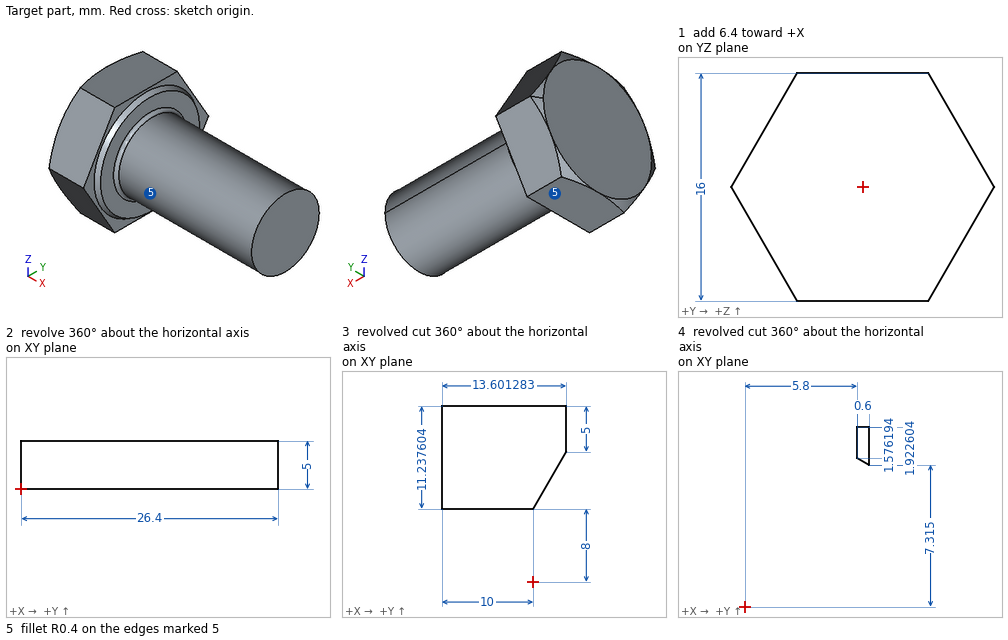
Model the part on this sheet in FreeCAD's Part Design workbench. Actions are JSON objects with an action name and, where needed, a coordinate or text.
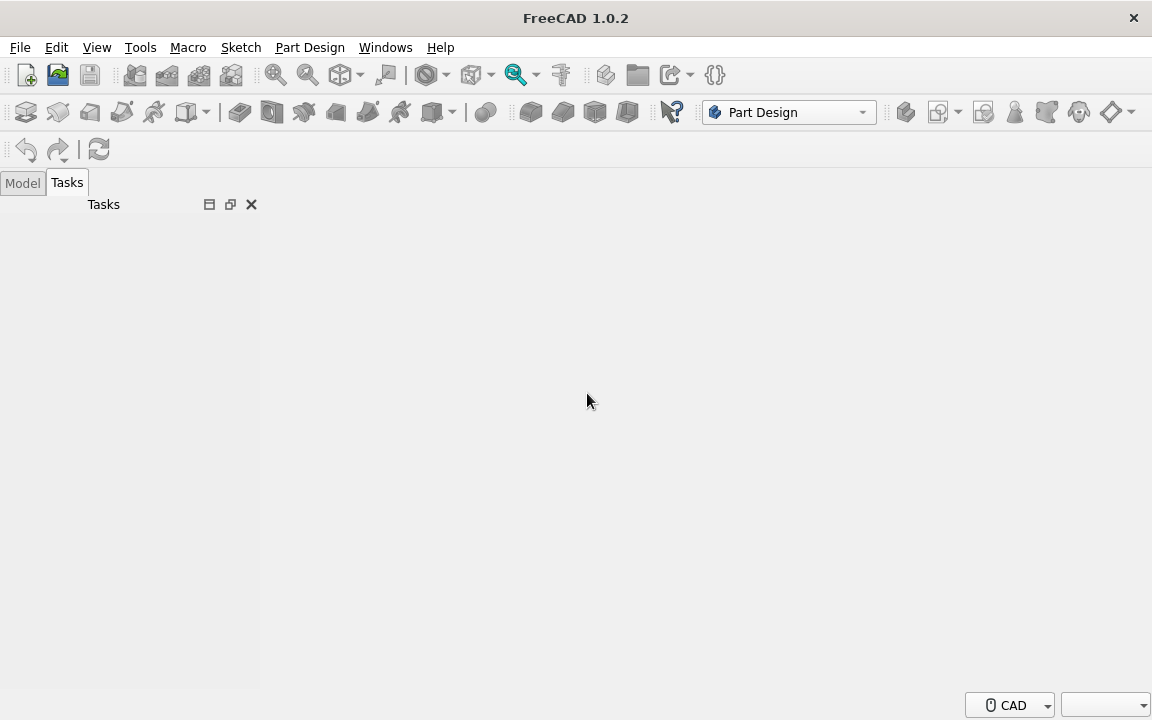
{"action": "left_click", "coordinate": [26, 76]}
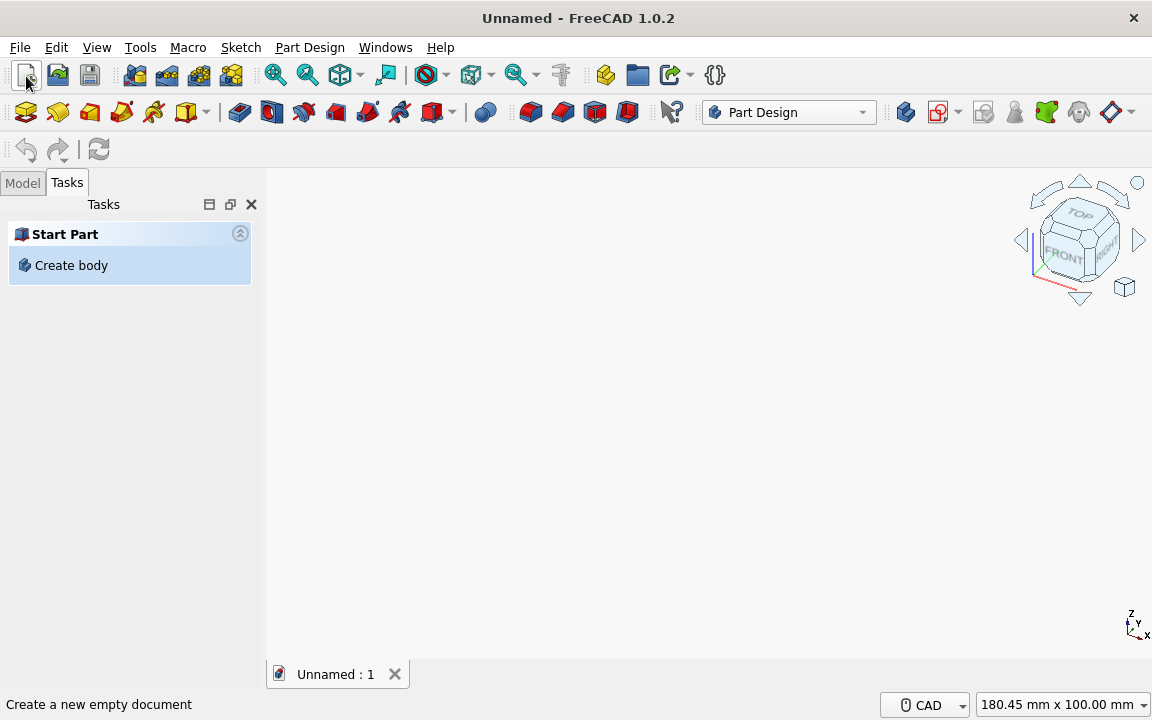
{"action": "left_click", "coordinate": [938, 112]}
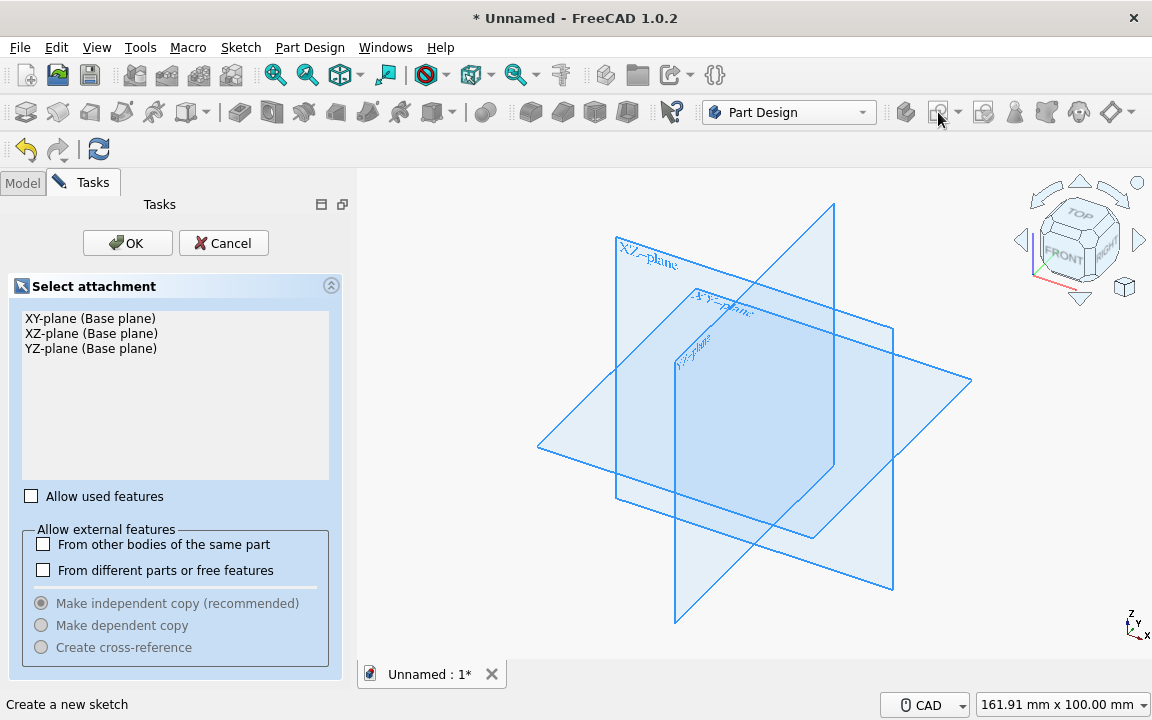
{"action": "left_click", "coordinate": [82, 348]}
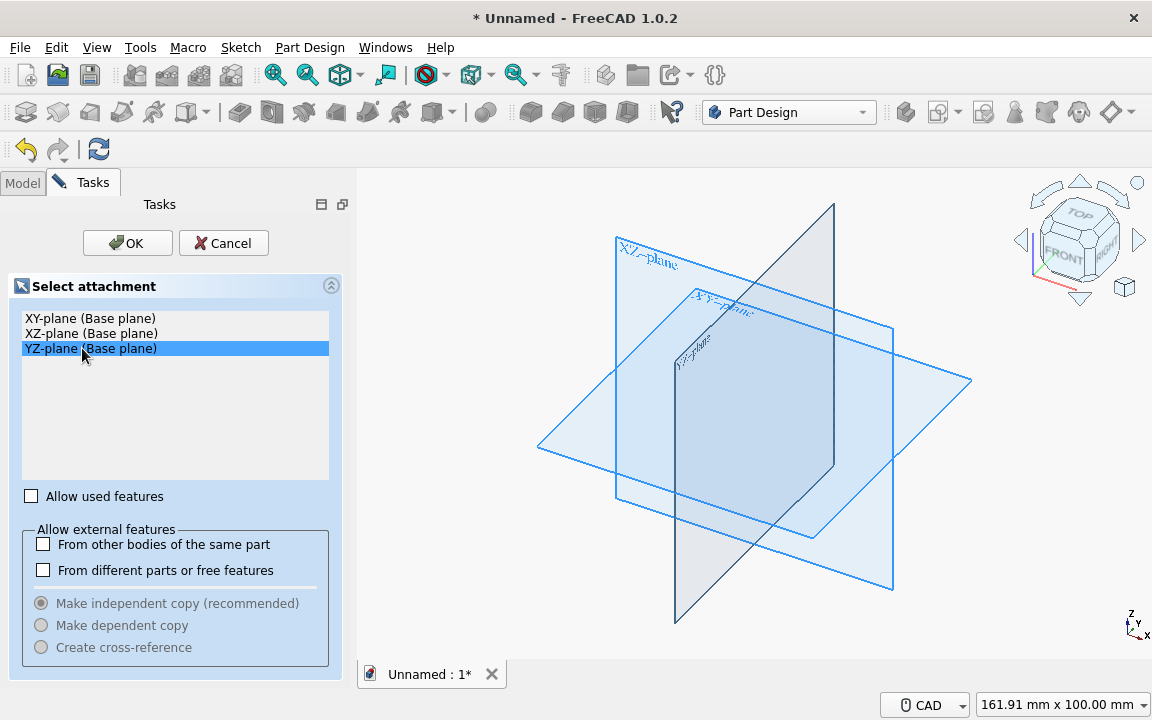
{"action": "left_click", "coordinate": [128, 243]}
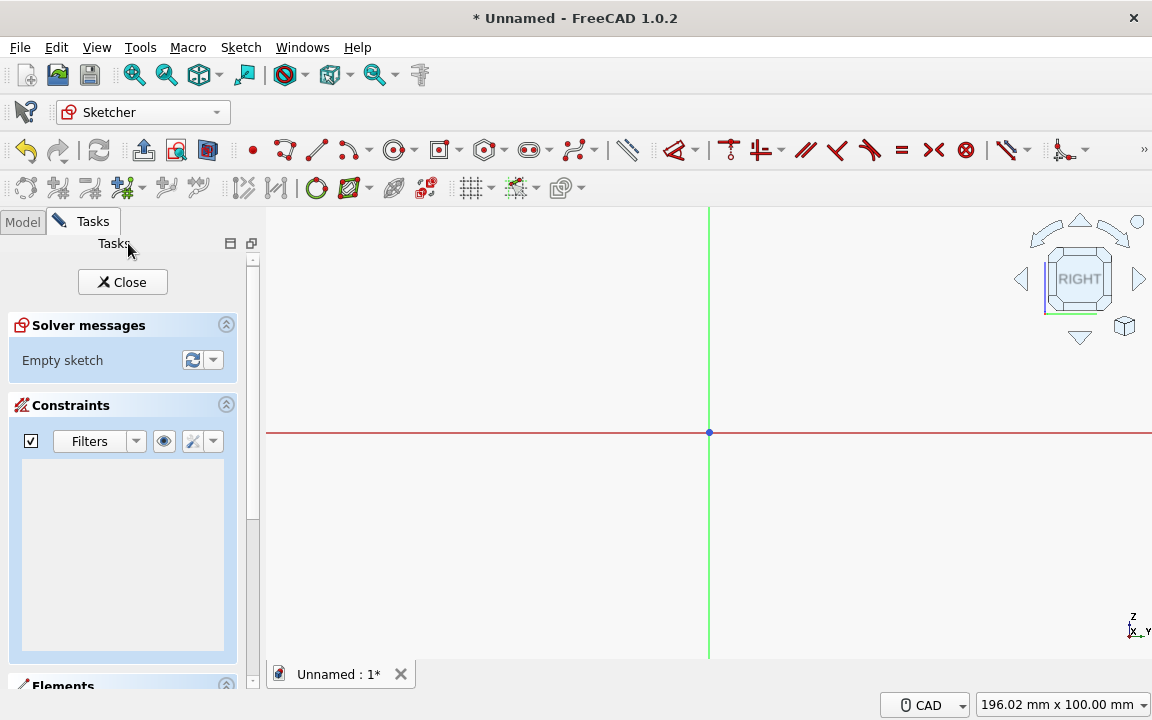
{"action": "scroll", "coordinate": [731, 433], "scroll_direction": "up", "scroll_amount": 7}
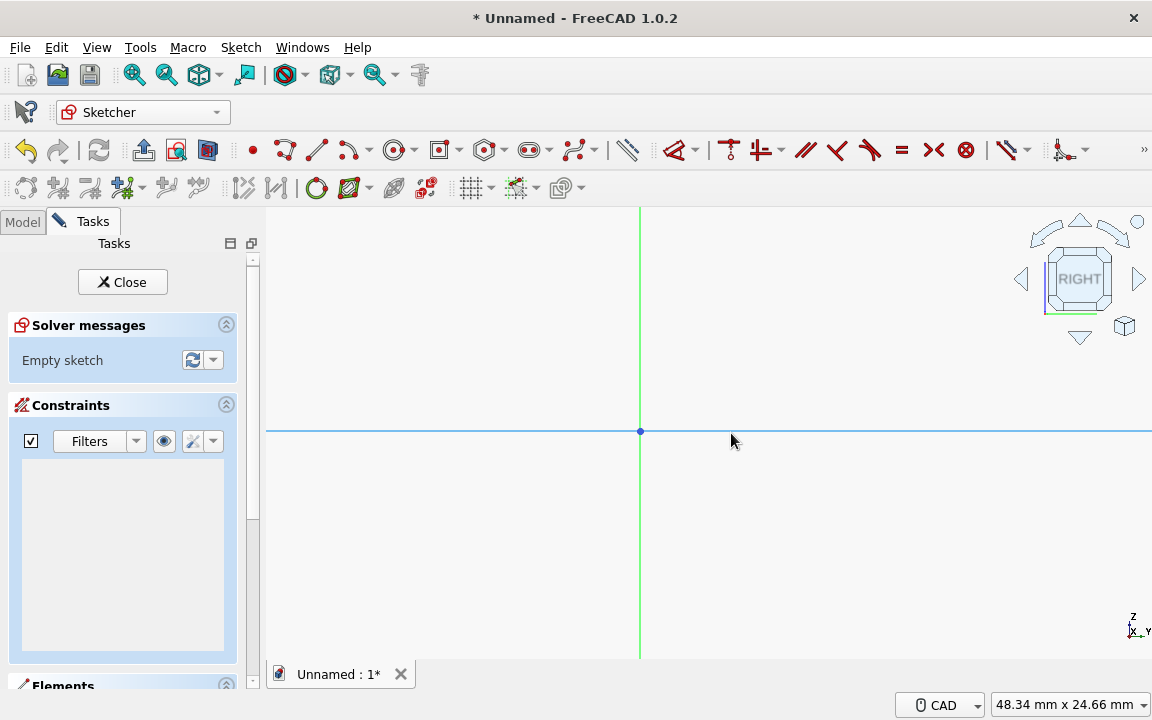
{"action": "left_click", "coordinate": [484, 150]}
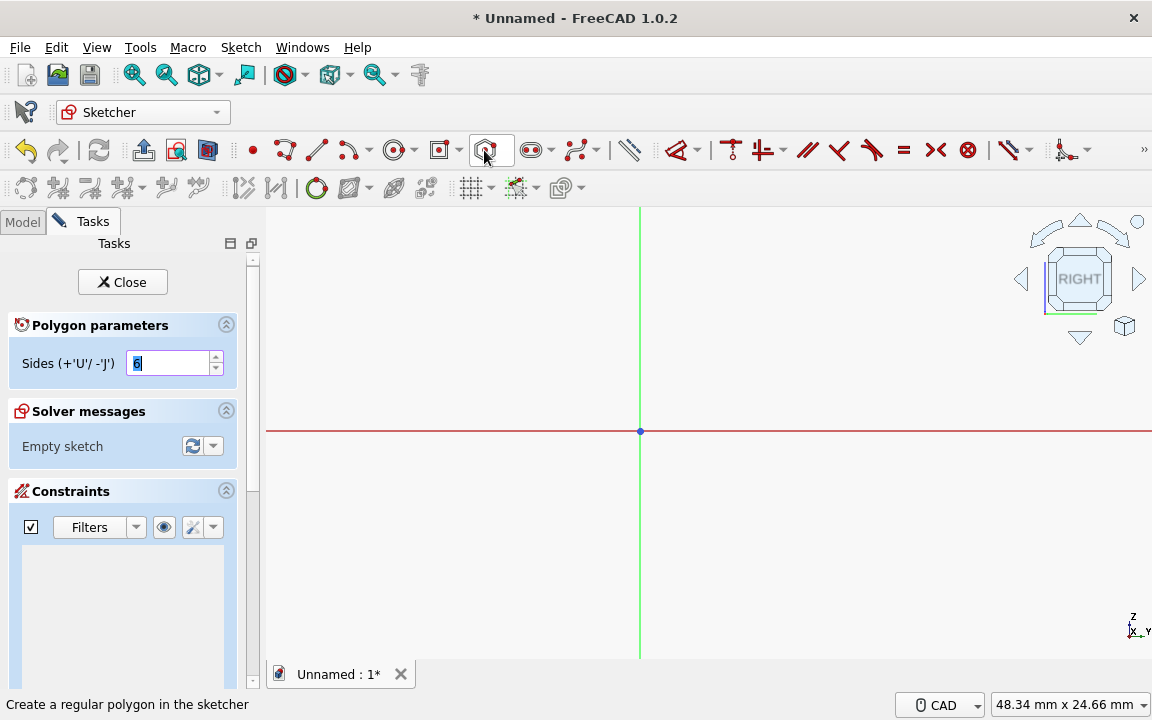
{"action": "left_click", "coordinate": [640, 431]}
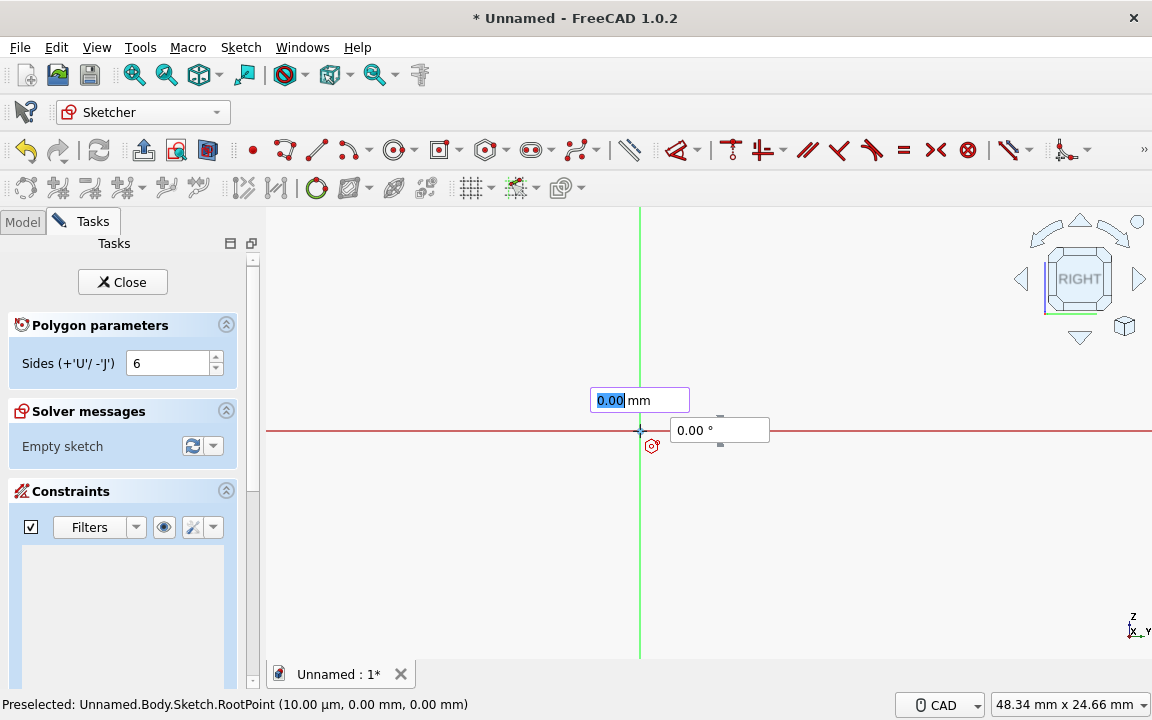
{"action": "left_click", "coordinate": [810, 431]}
{"action": "right_click", "coordinate": [810, 431]}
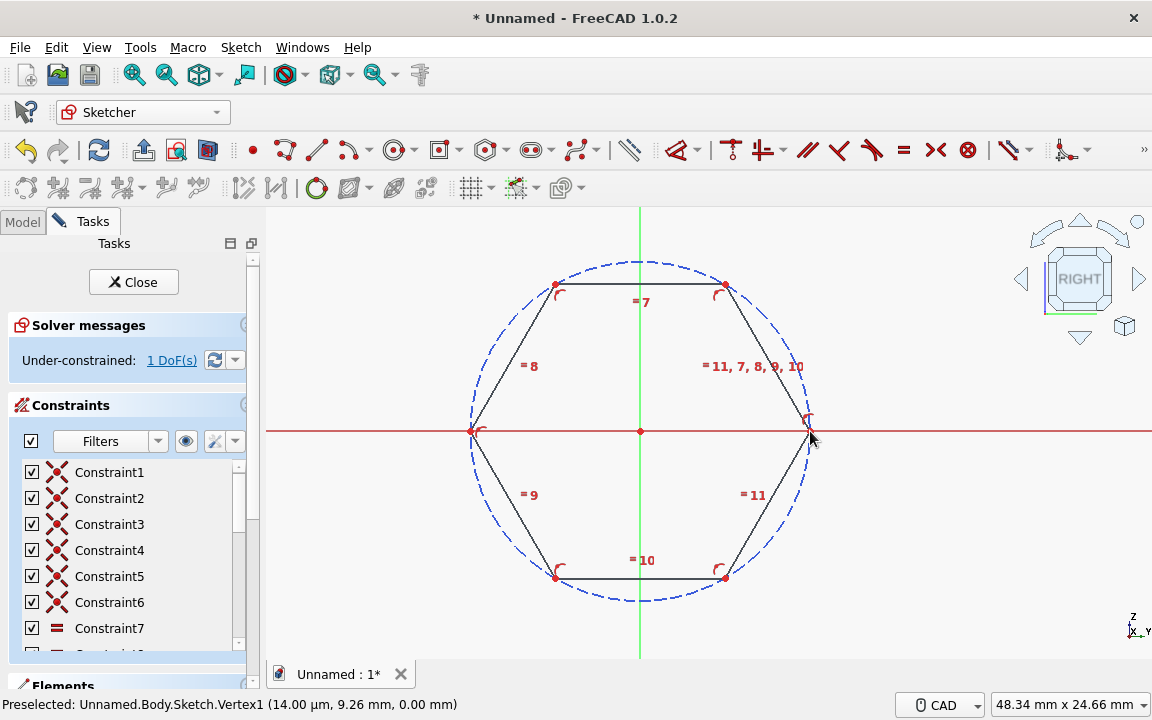
{"action": "left_click", "coordinate": [676, 150]}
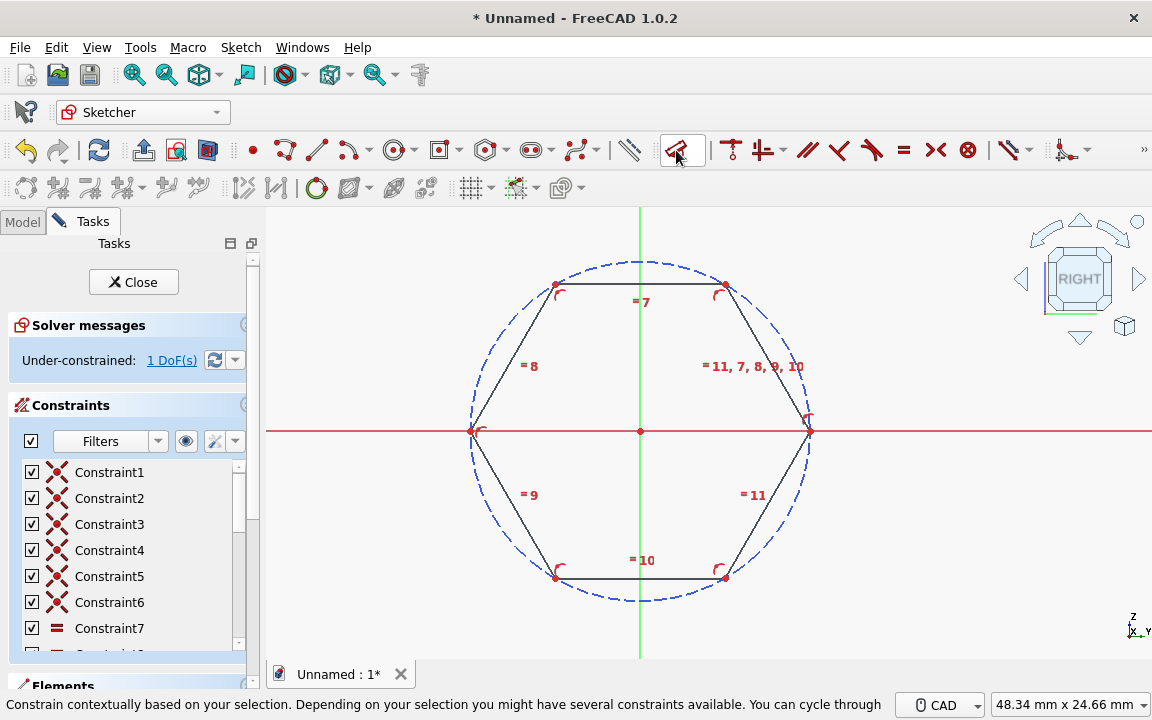
{"action": "left_click", "coordinate": [555, 579]}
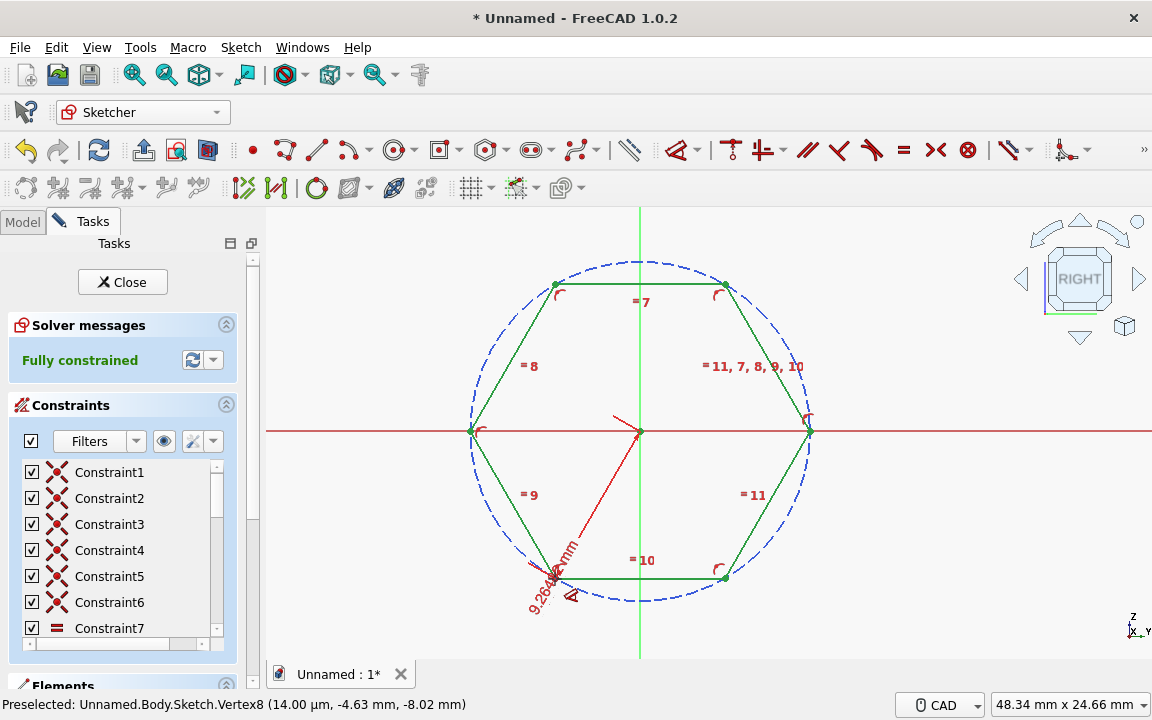
{"action": "left_click", "coordinate": [725, 284]}
{"action": "left_click", "coordinate": [807, 329]}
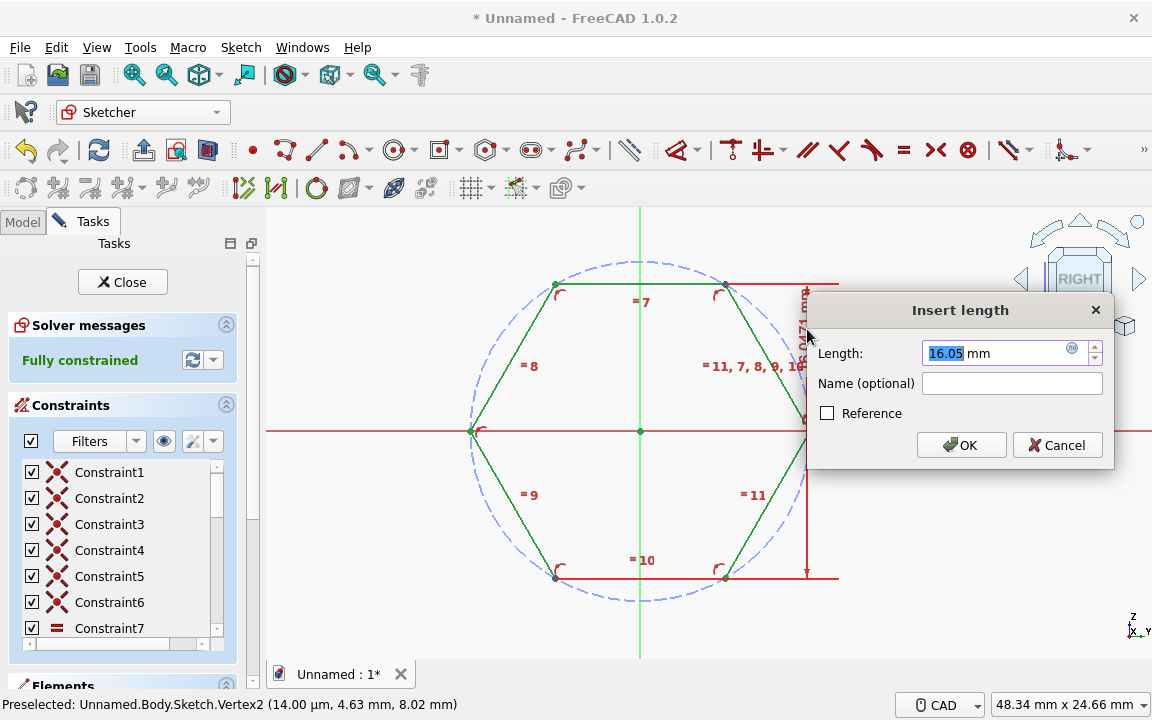
{"action": "type", "text": "16"}
{"action": "key", "text": "Return"}
{"action": "key", "text": "Escape"}